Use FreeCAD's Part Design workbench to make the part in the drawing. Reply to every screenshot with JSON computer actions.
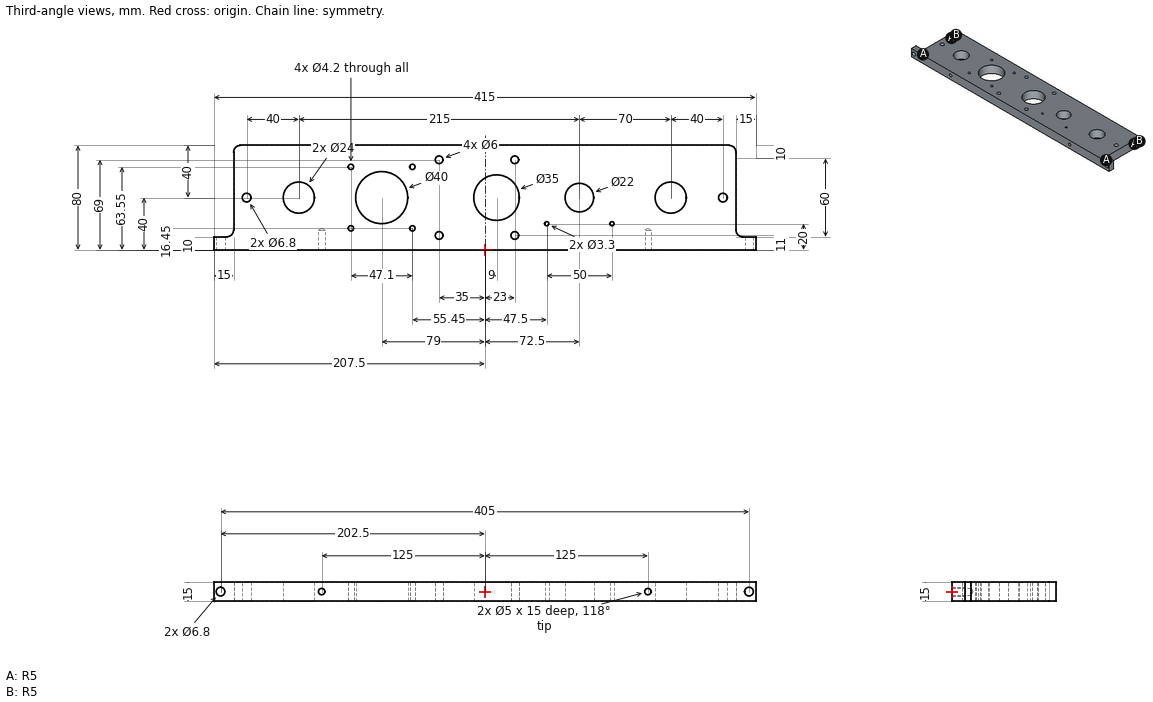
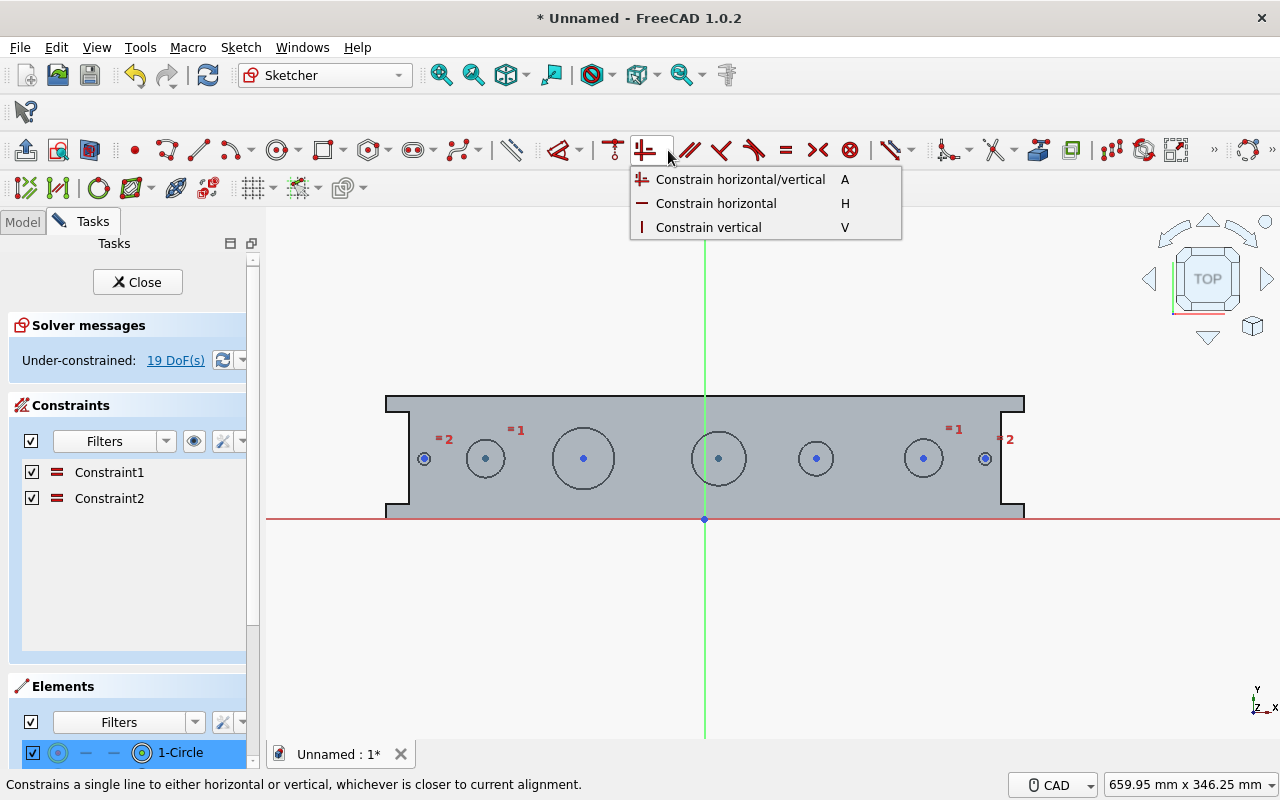
{"action": "left_click", "coordinate": [766, 203]}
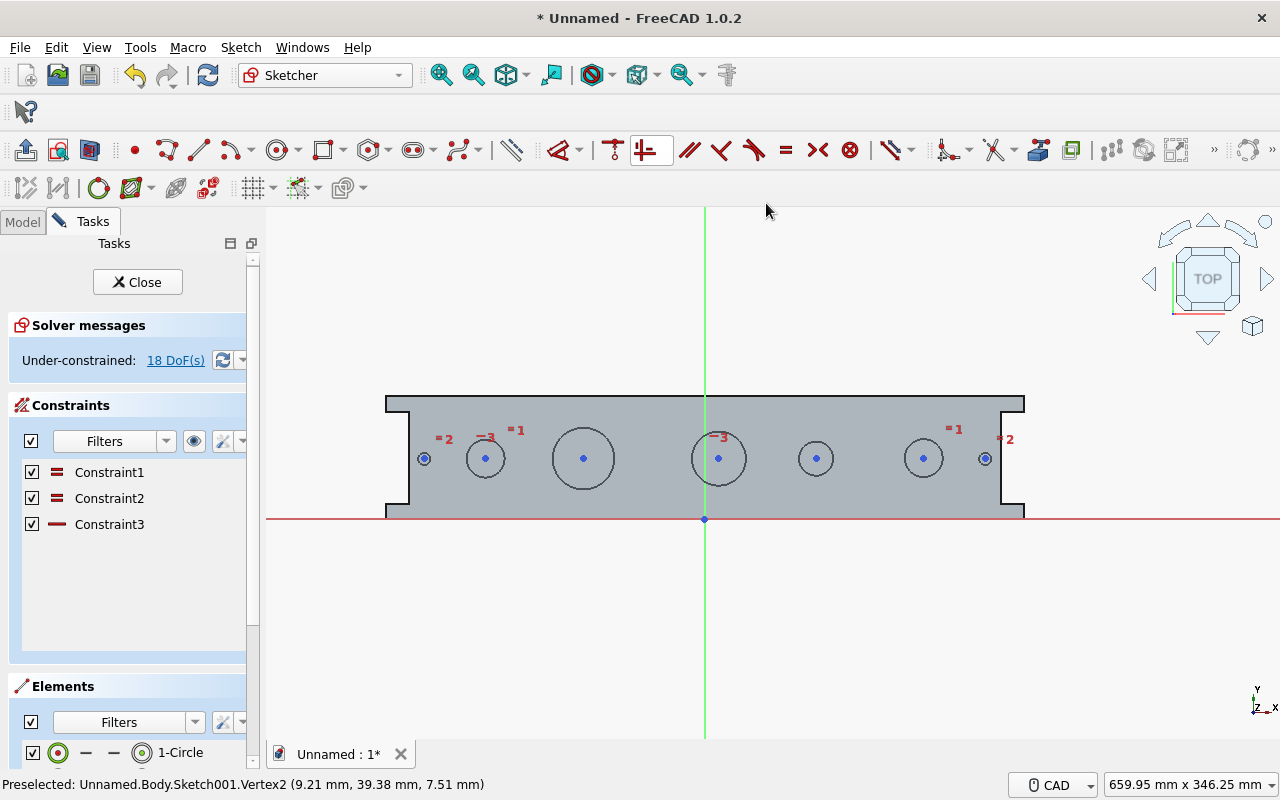
{"action": "left_click", "coordinate": [719, 459]}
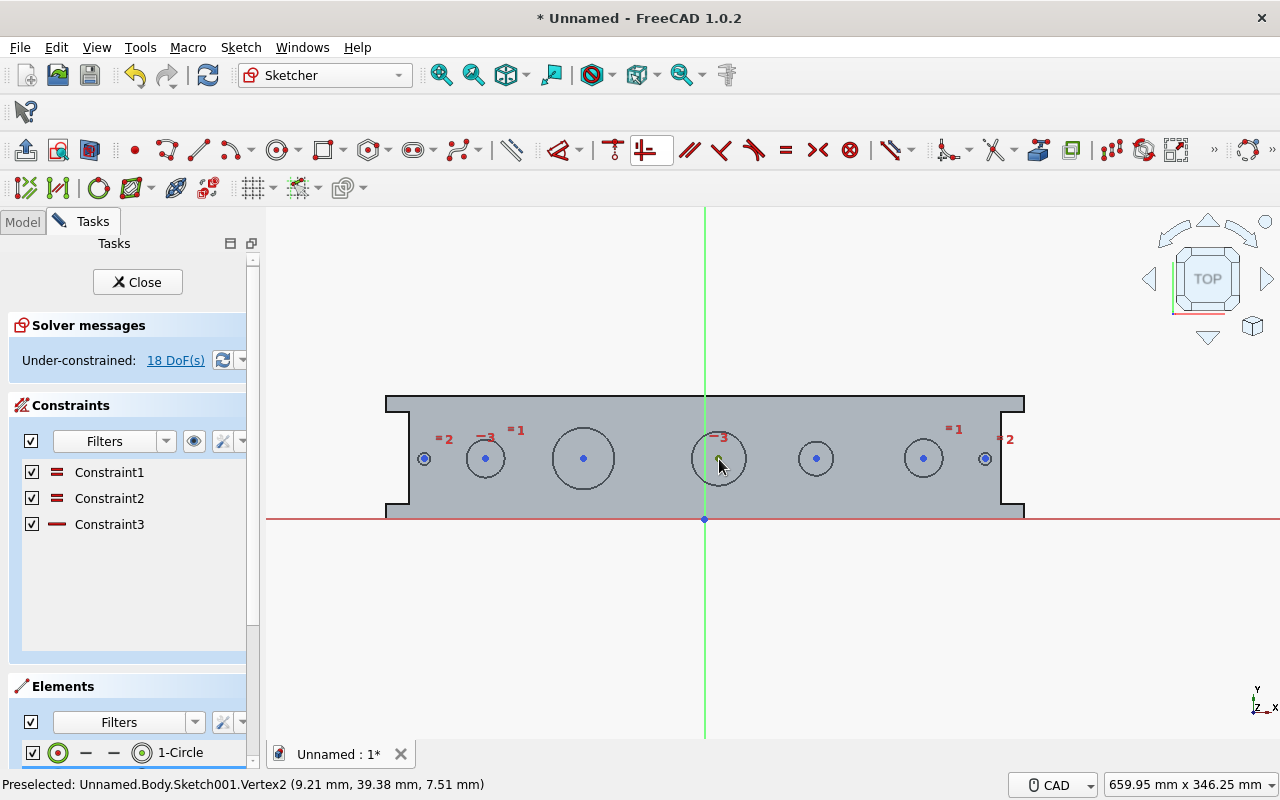
{"action": "left_click", "coordinate": [816, 459]}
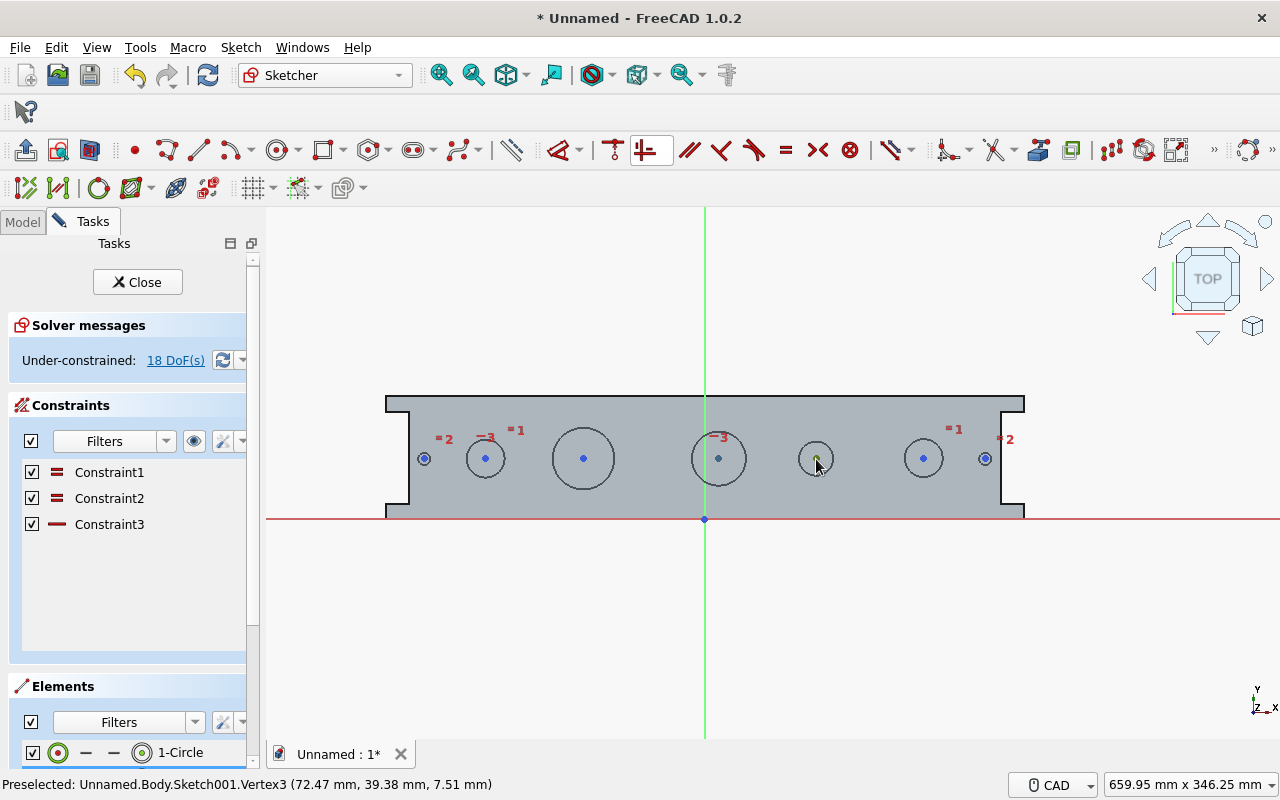
{"action": "key", "text": "h"}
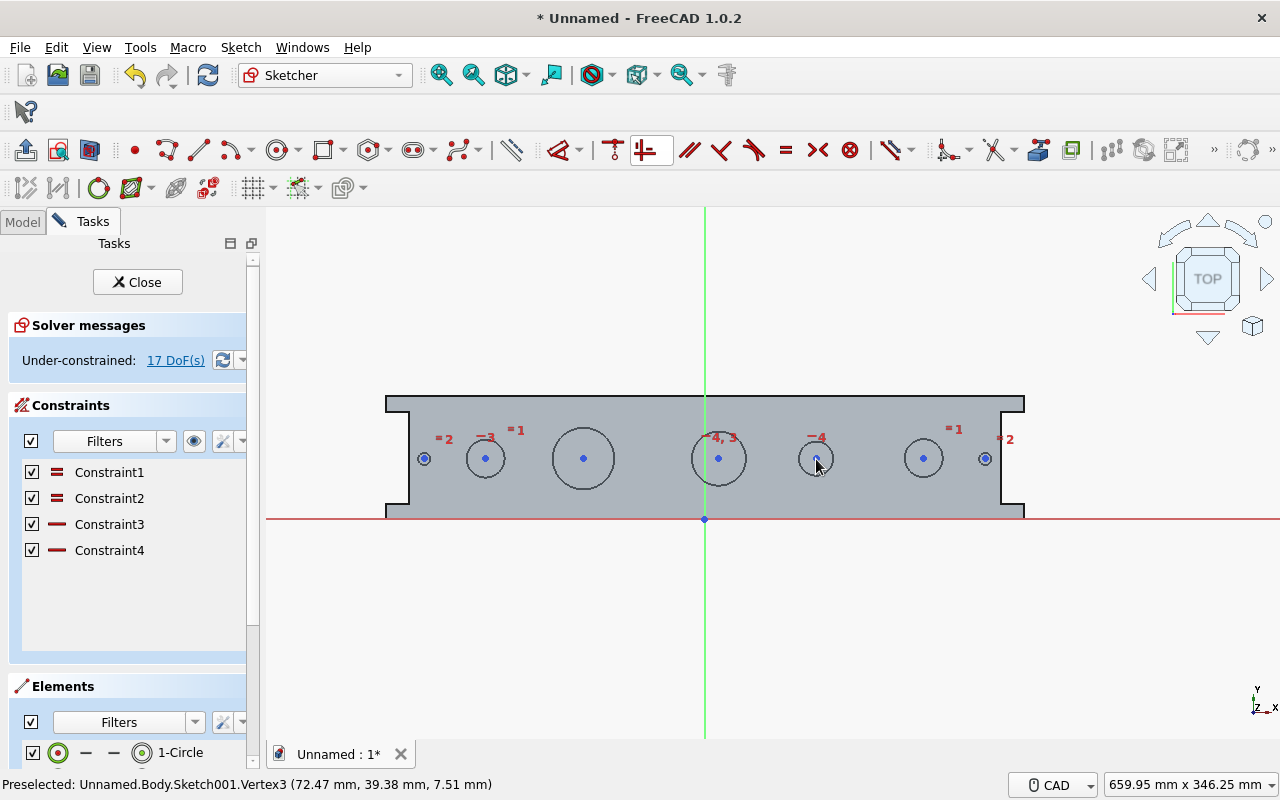
{"action": "left_click", "coordinate": [486, 459]}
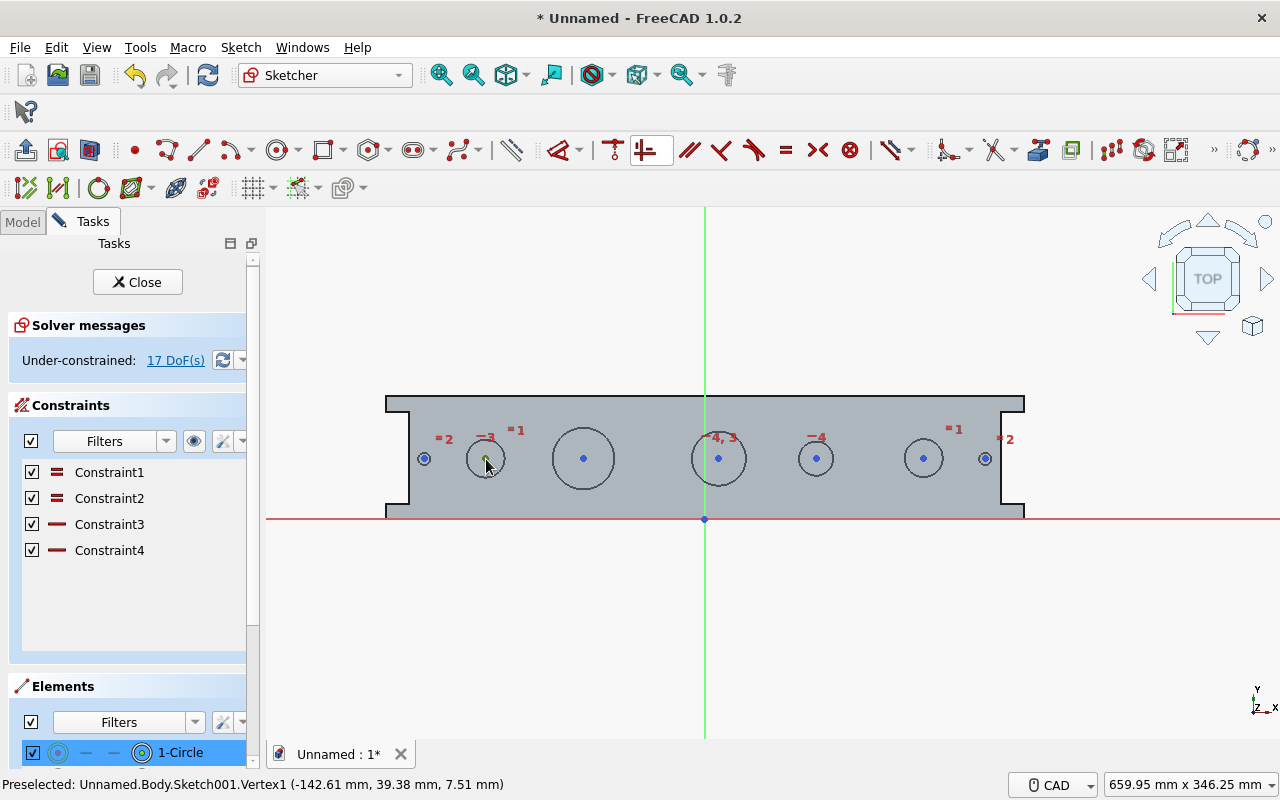
{"action": "left_click", "coordinate": [583, 459]}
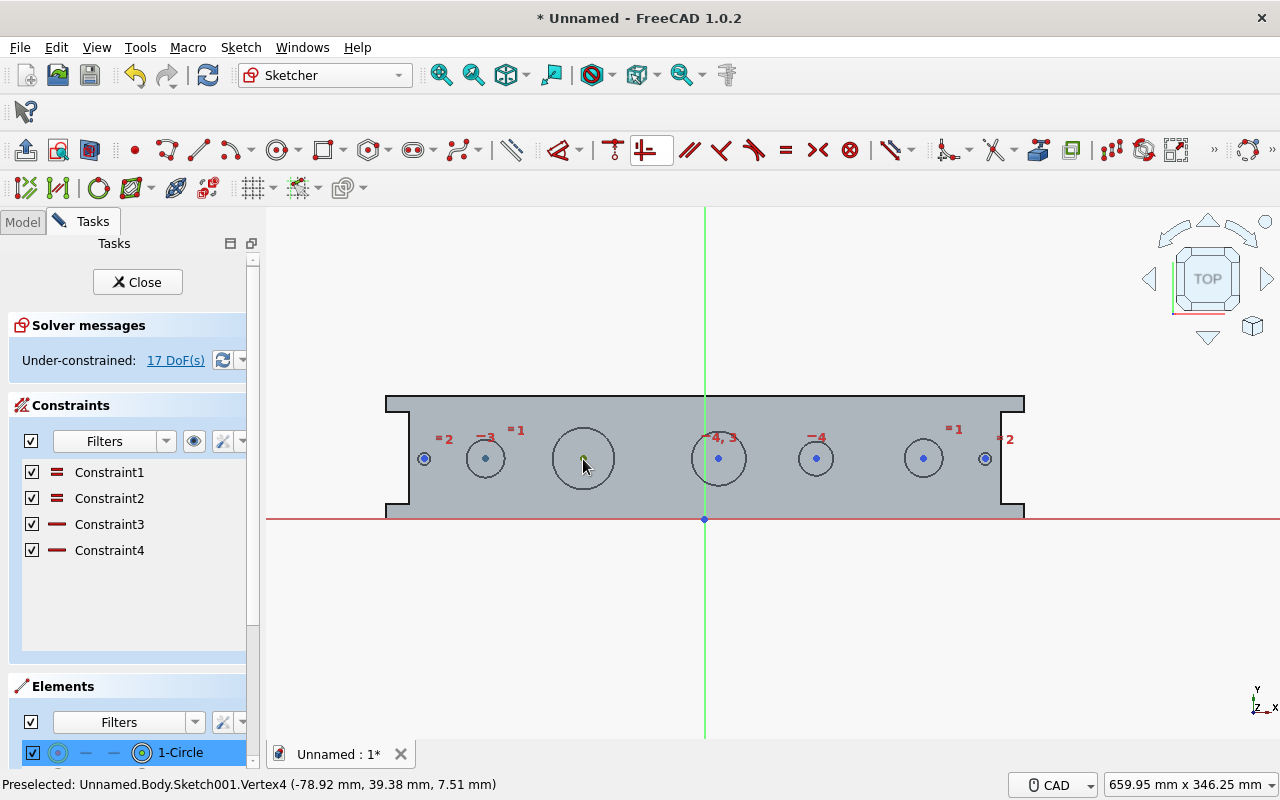
{"action": "left_click", "coordinate": [668, 150]}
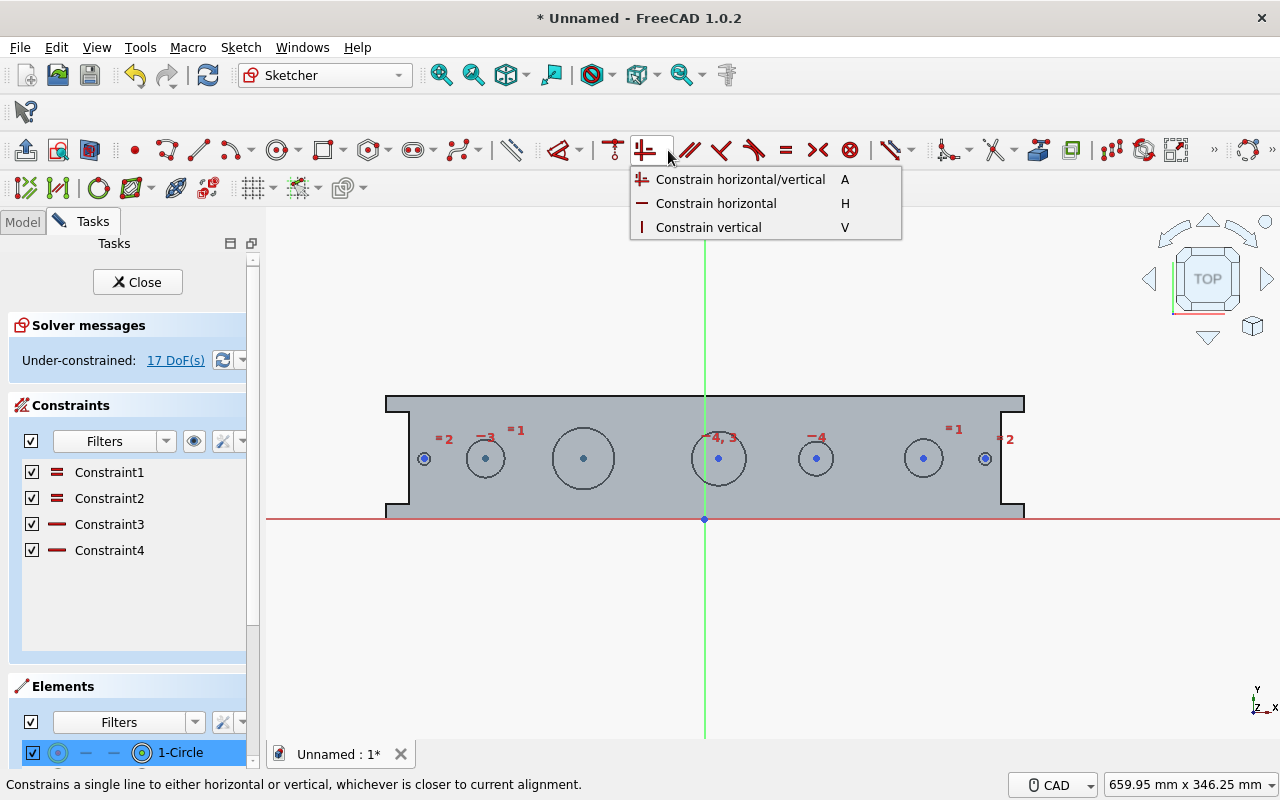
{"action": "left_click", "coordinate": [766, 203]}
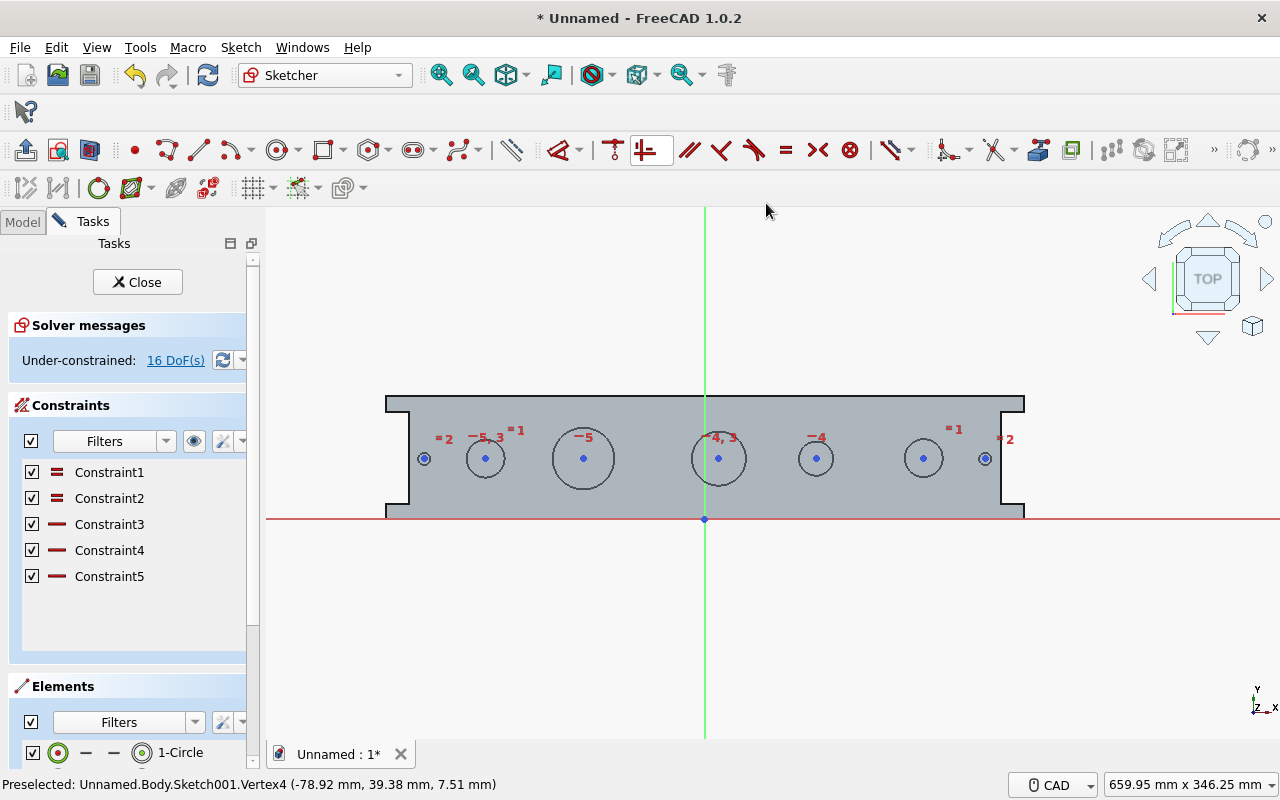
{"action": "left_click", "coordinate": [816, 459]}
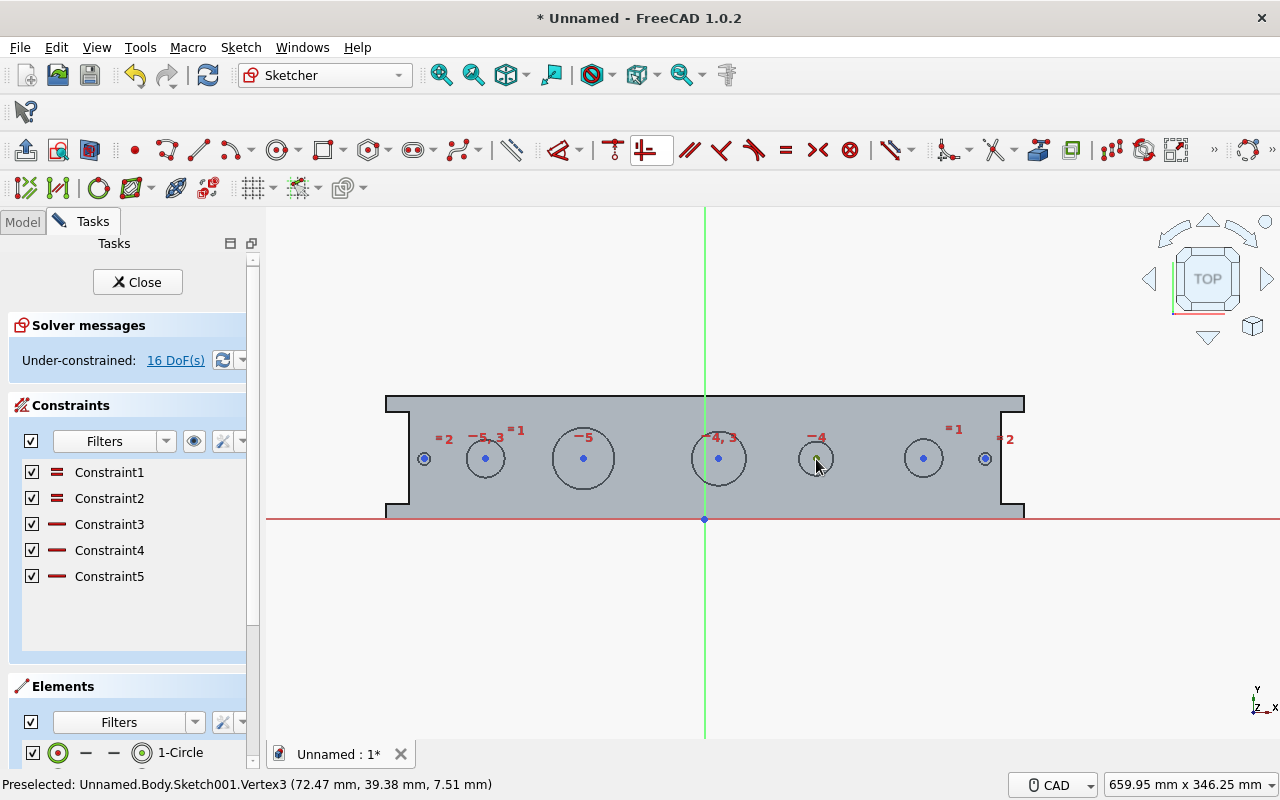
{"action": "left_click", "coordinate": [924, 458]}